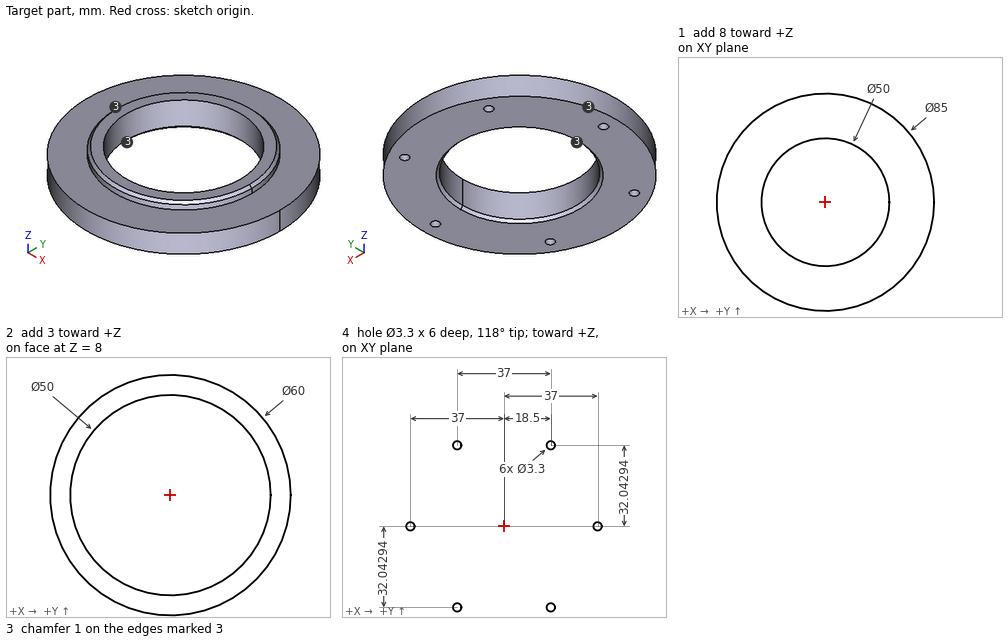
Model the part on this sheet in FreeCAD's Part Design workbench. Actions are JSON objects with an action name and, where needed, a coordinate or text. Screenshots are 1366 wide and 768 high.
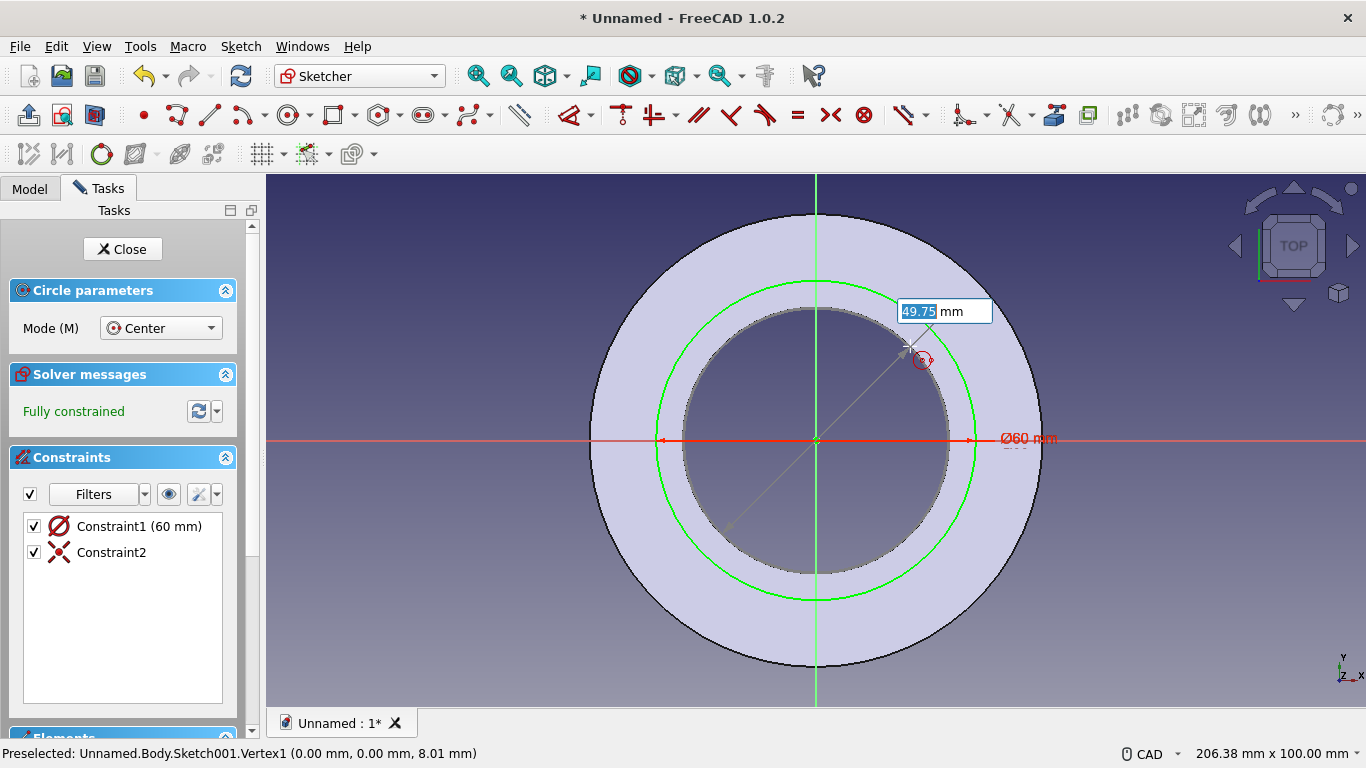
{"action": "type", "text": "50"}
{"action": "key", "text": "Return"}
{"action": "key", "text": "Escape"}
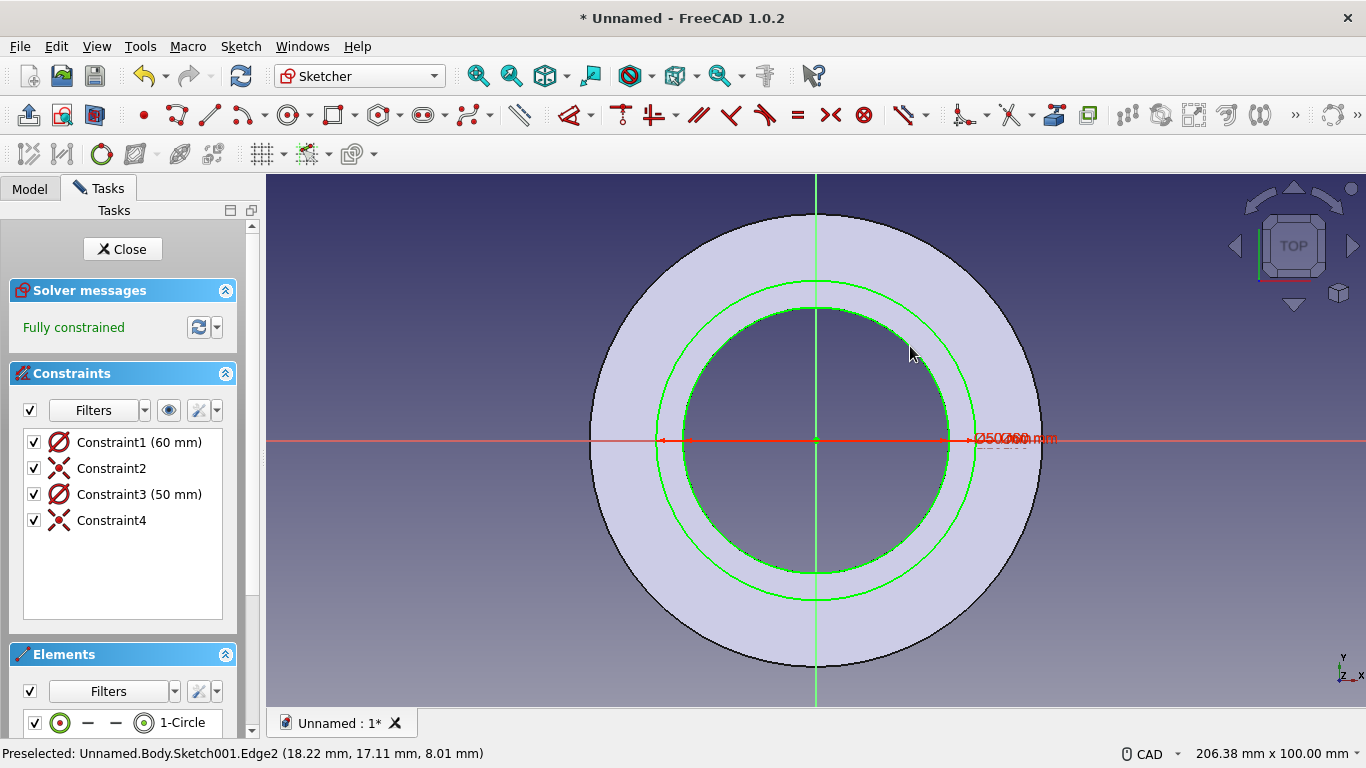
{"action": "left_click", "coordinate": [123, 249]}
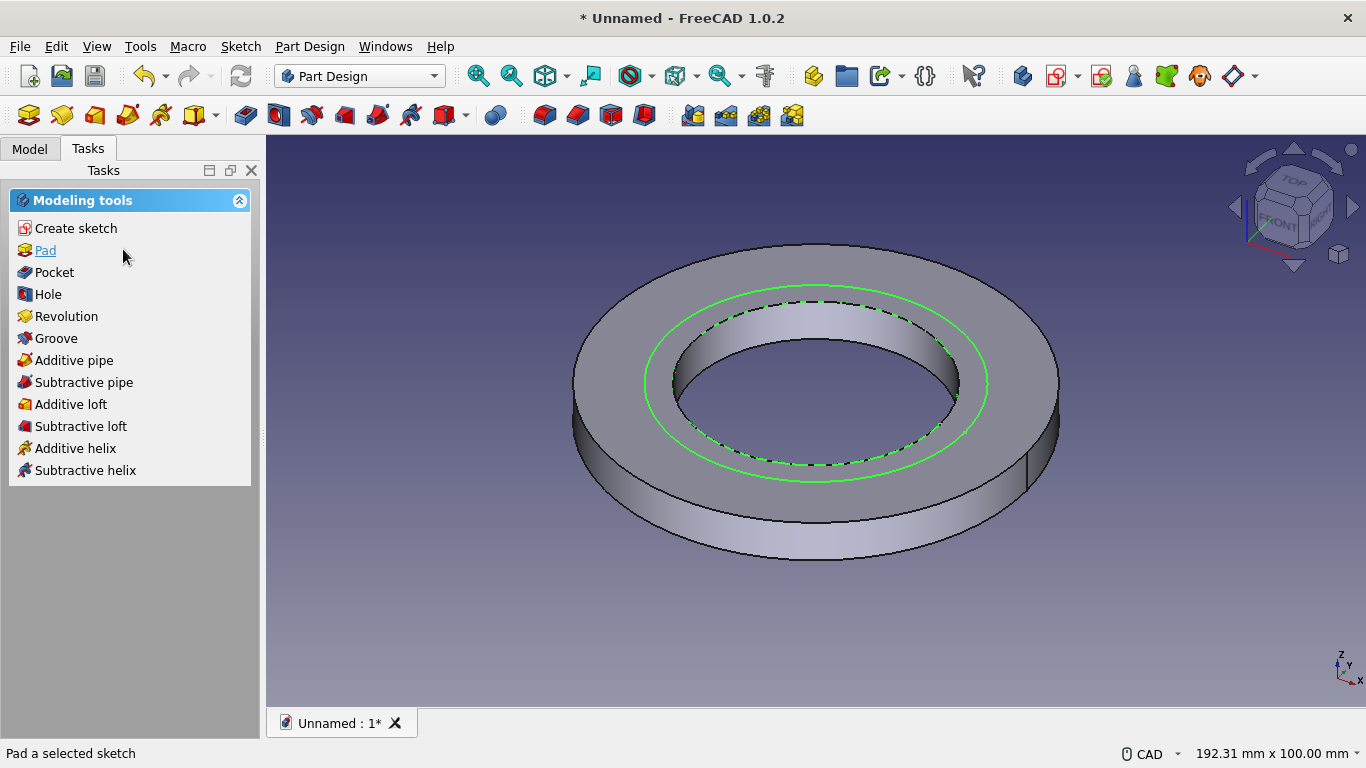
{"action": "left_click", "coordinate": [29, 116]}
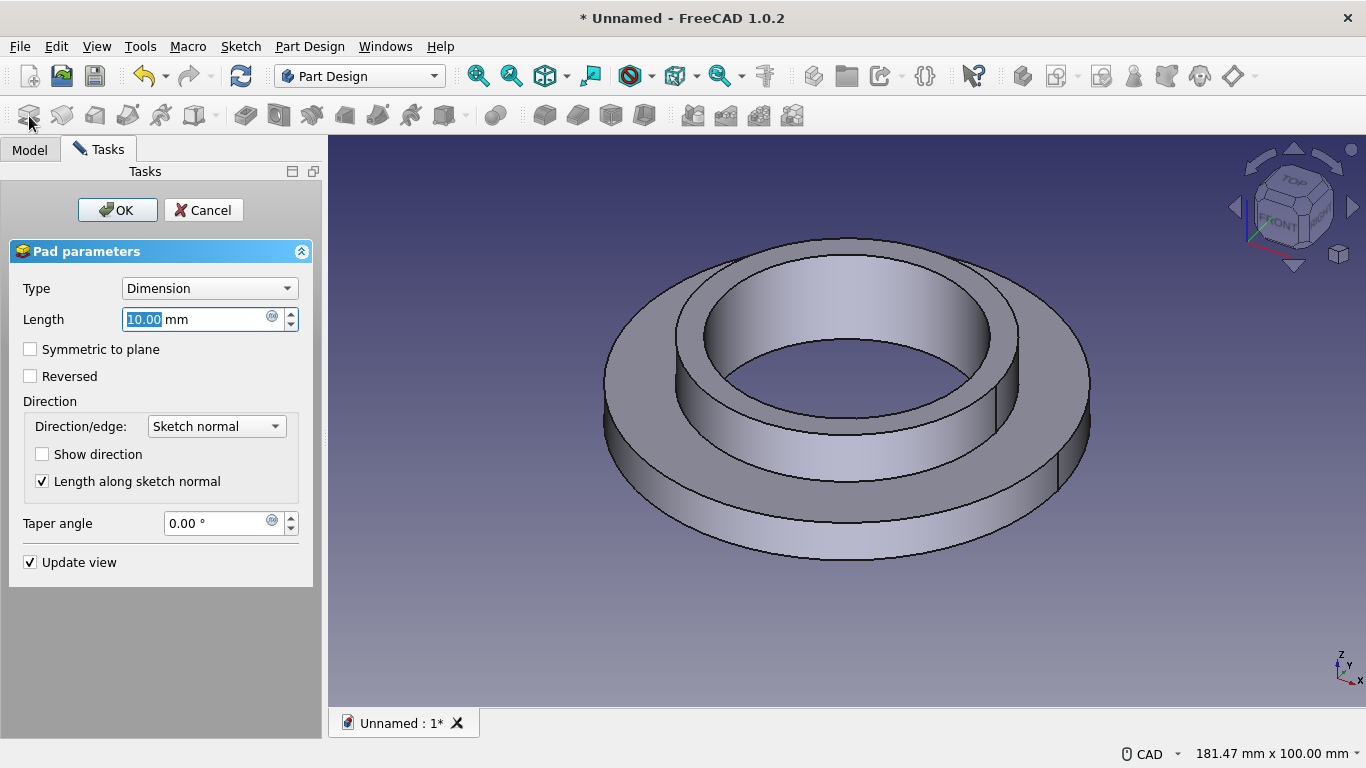
{"action": "type", "text": "3"}
{"action": "key", "text": "Tab"}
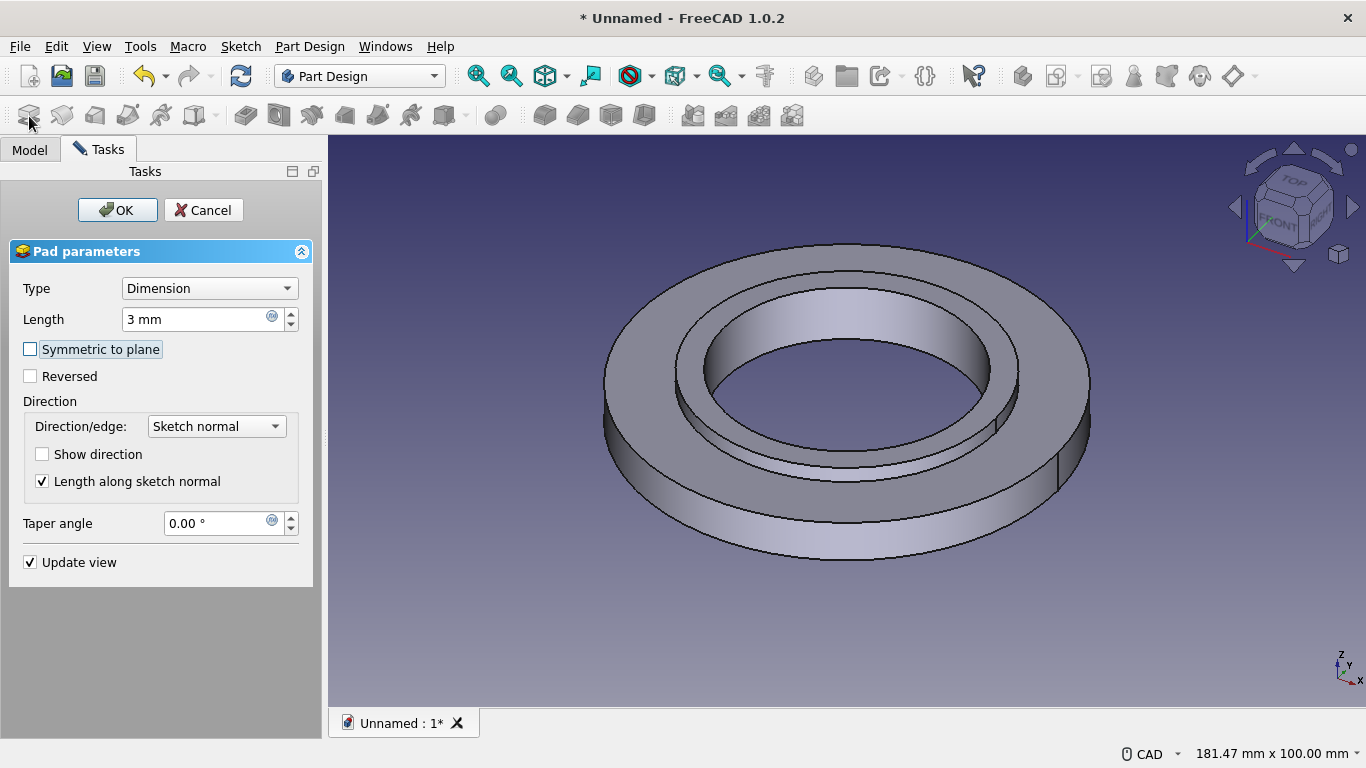
{"action": "left_click", "coordinate": [118, 210]}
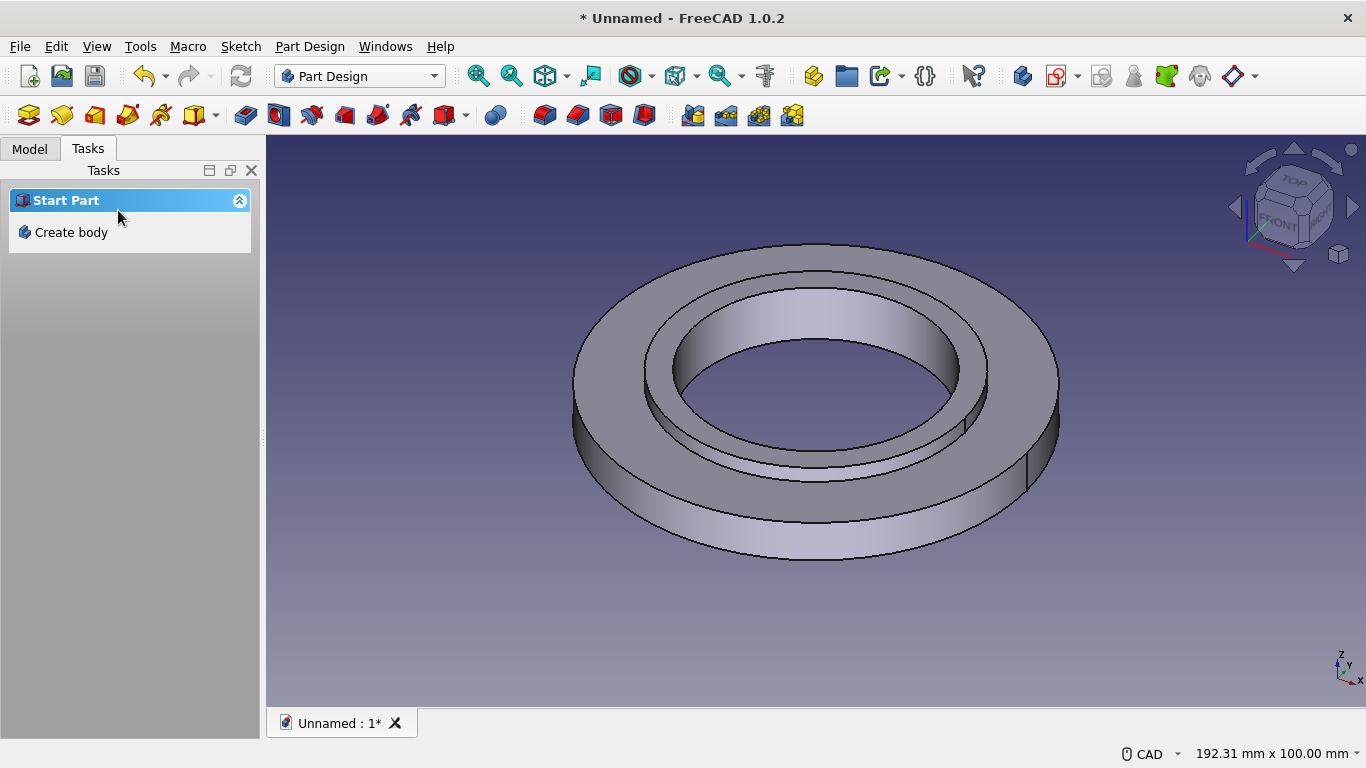
{"action": "left_click", "coordinate": [645, 379]}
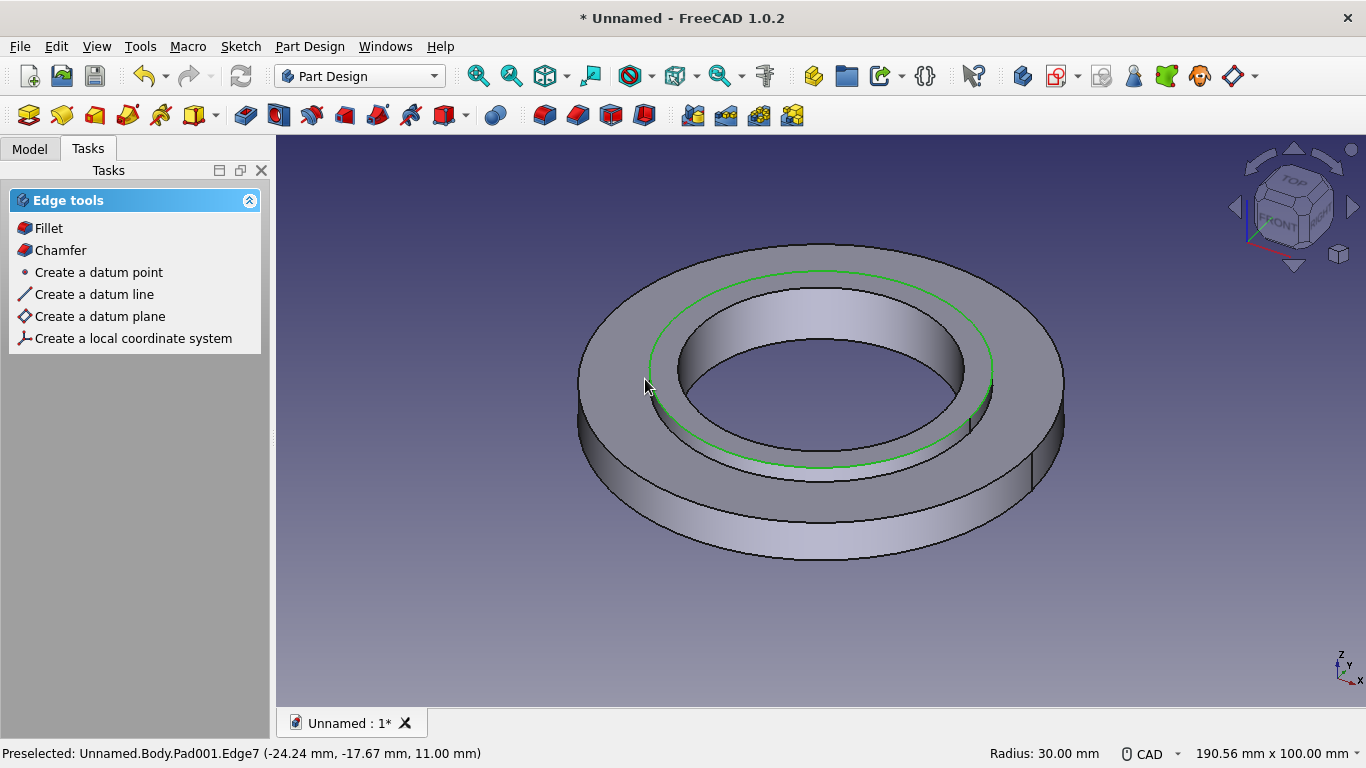
{"action": "key", "text": "0"}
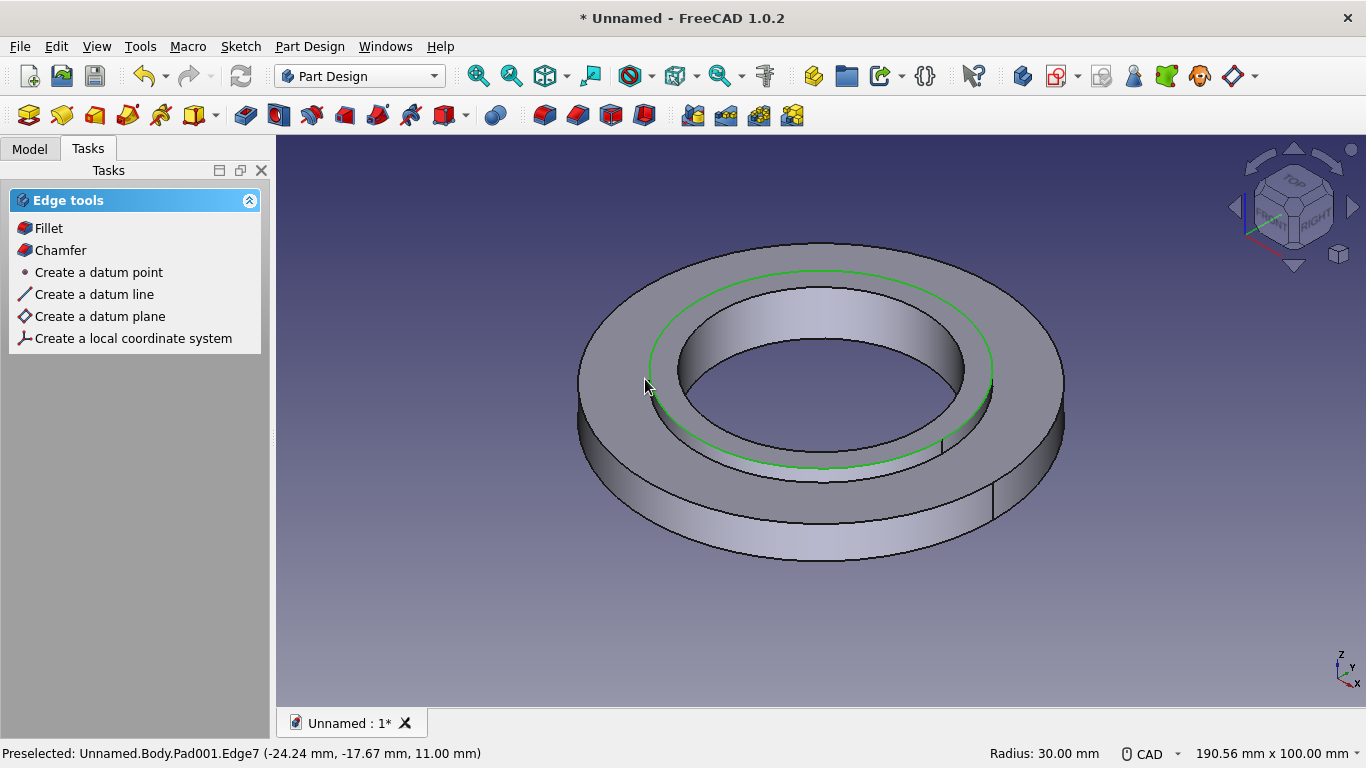
{"action": "left_click", "coordinate": [948, 383], "text": "ctrl"}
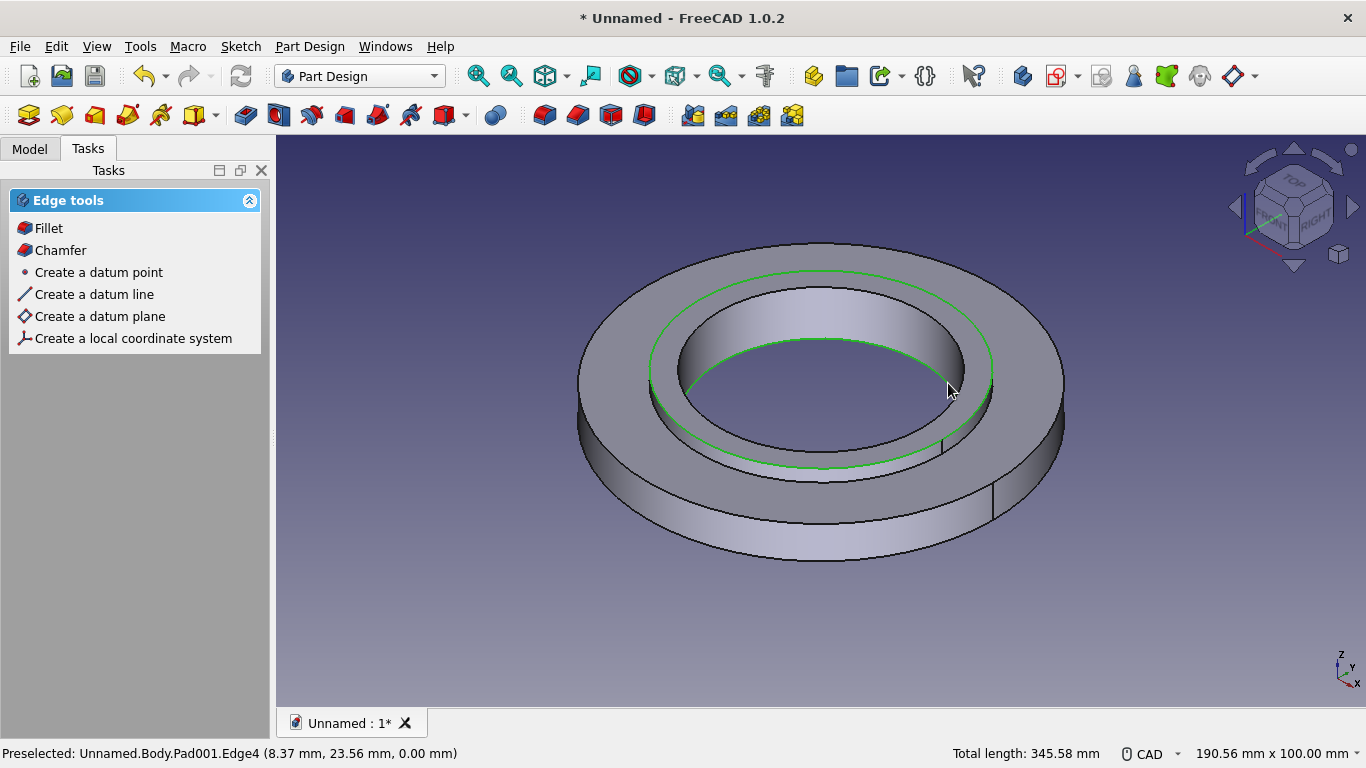
{"action": "left_click", "coordinate": [578, 116]}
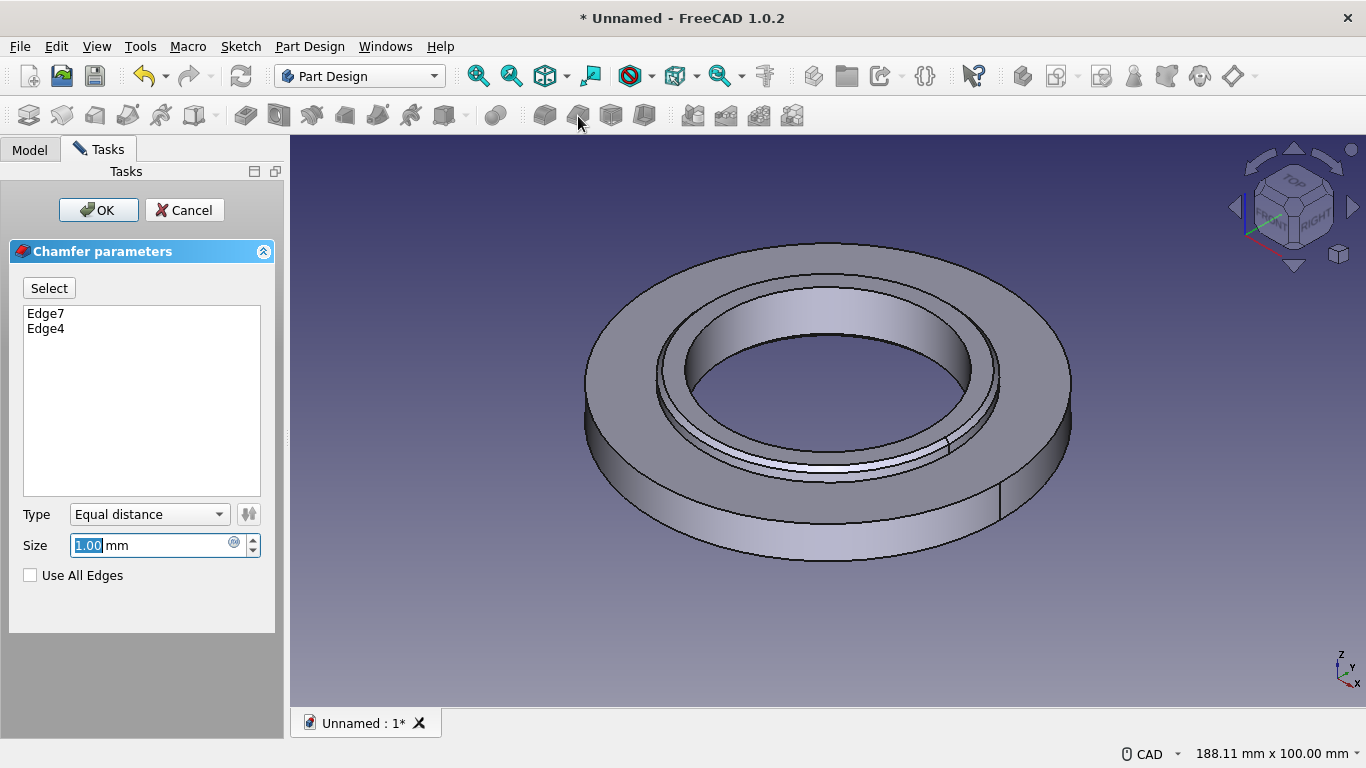
{"action": "type", "text": "1"}
{"action": "key", "text": "Tab"}